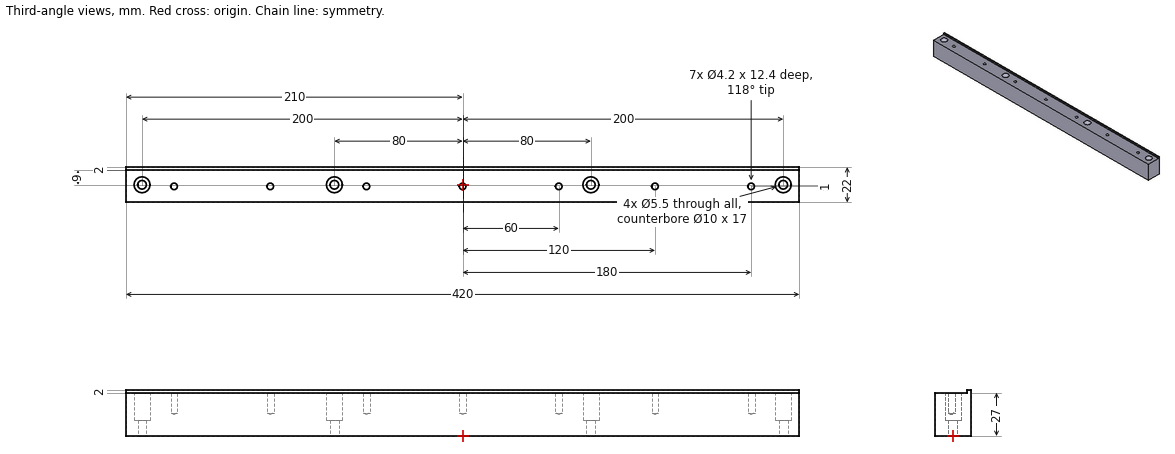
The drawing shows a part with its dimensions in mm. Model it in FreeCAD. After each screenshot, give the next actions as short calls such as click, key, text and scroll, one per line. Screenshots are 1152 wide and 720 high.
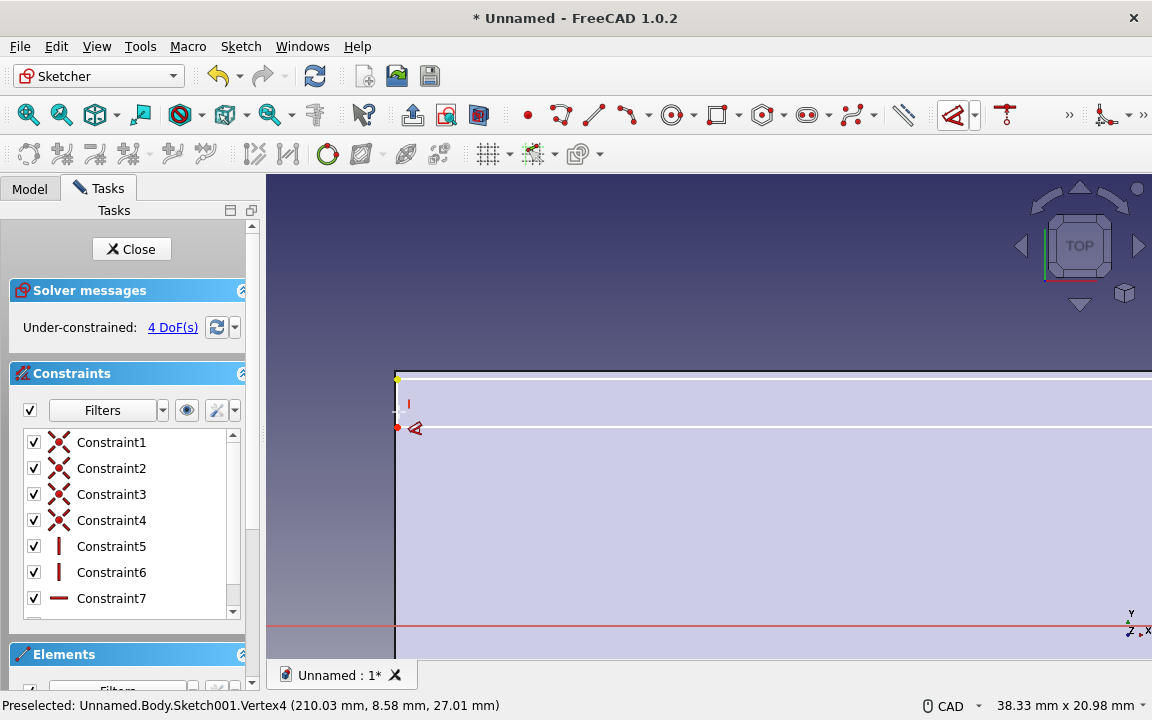
click(397, 403)
click(363, 403)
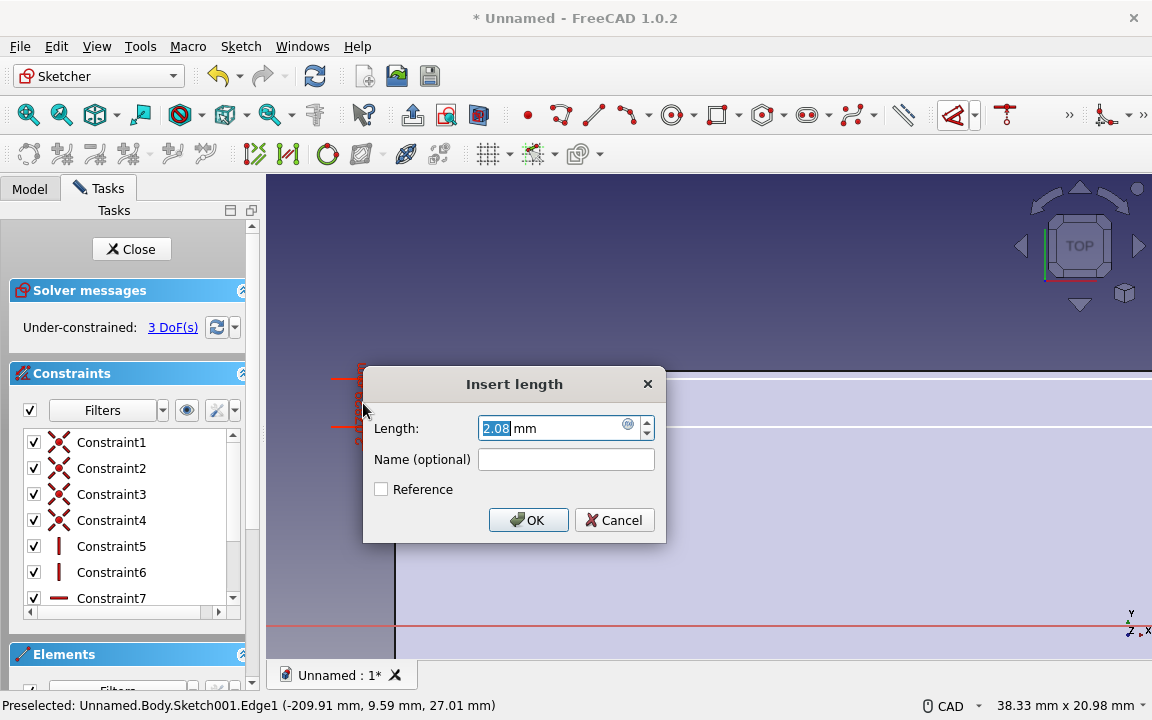
text(2)
key(Return)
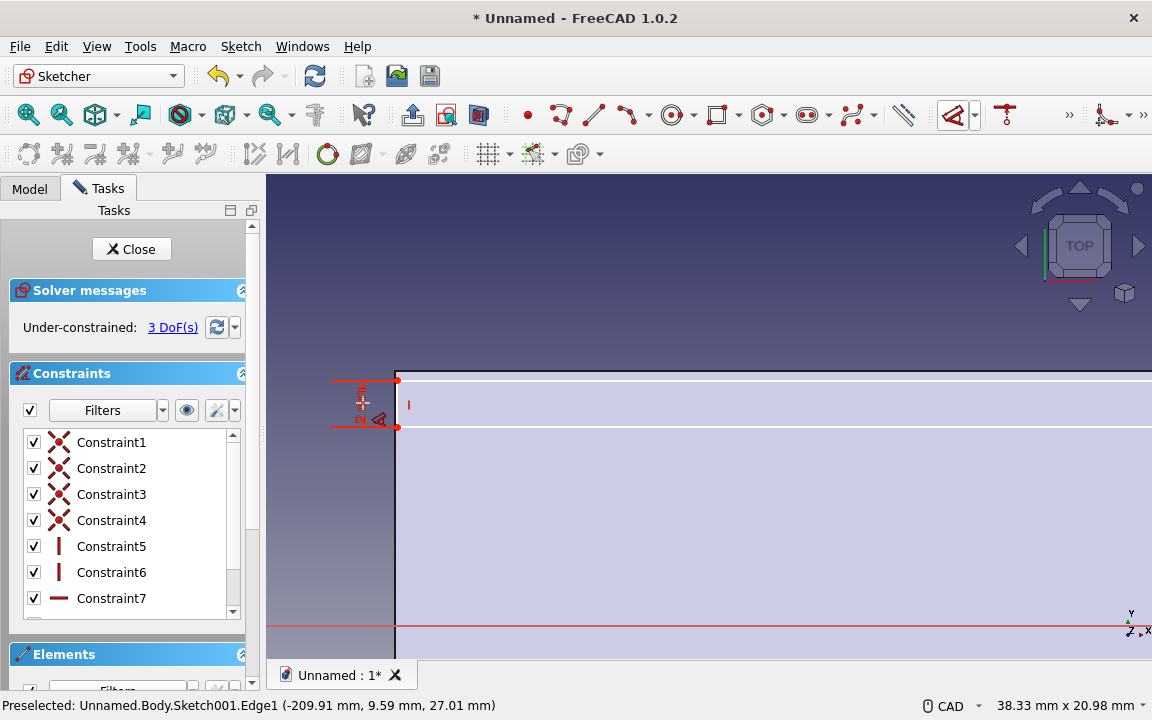
scroll(399, 412, down, 15)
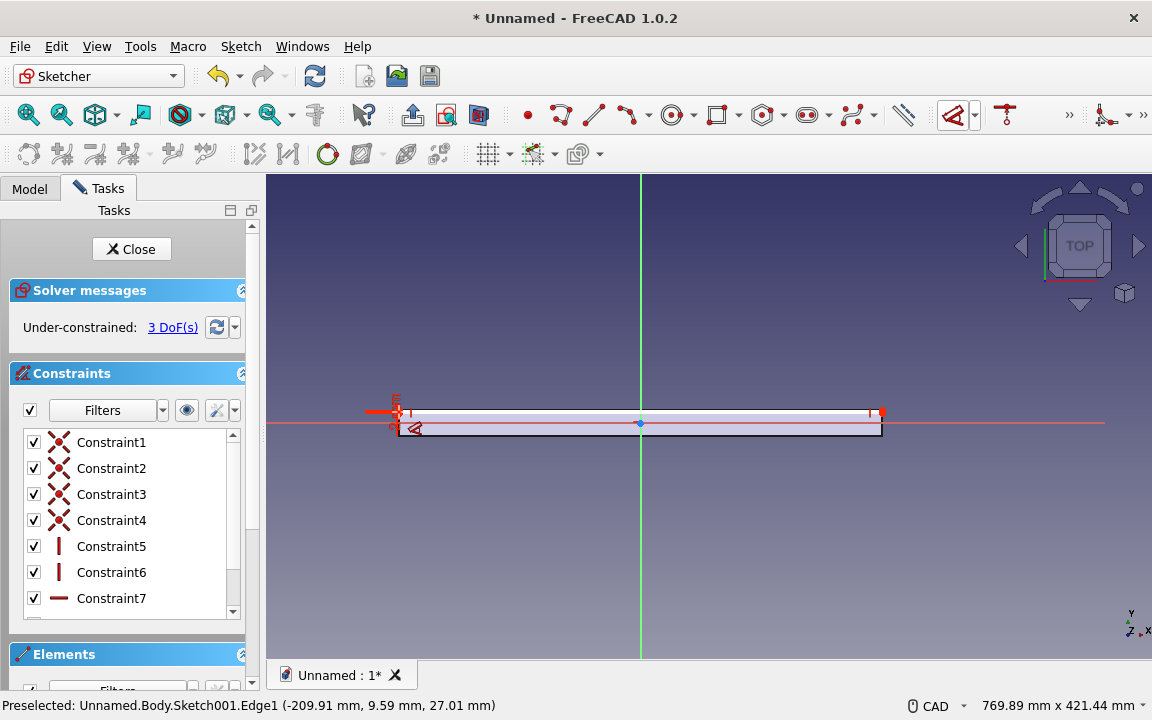
scroll(399, 413, up, 9)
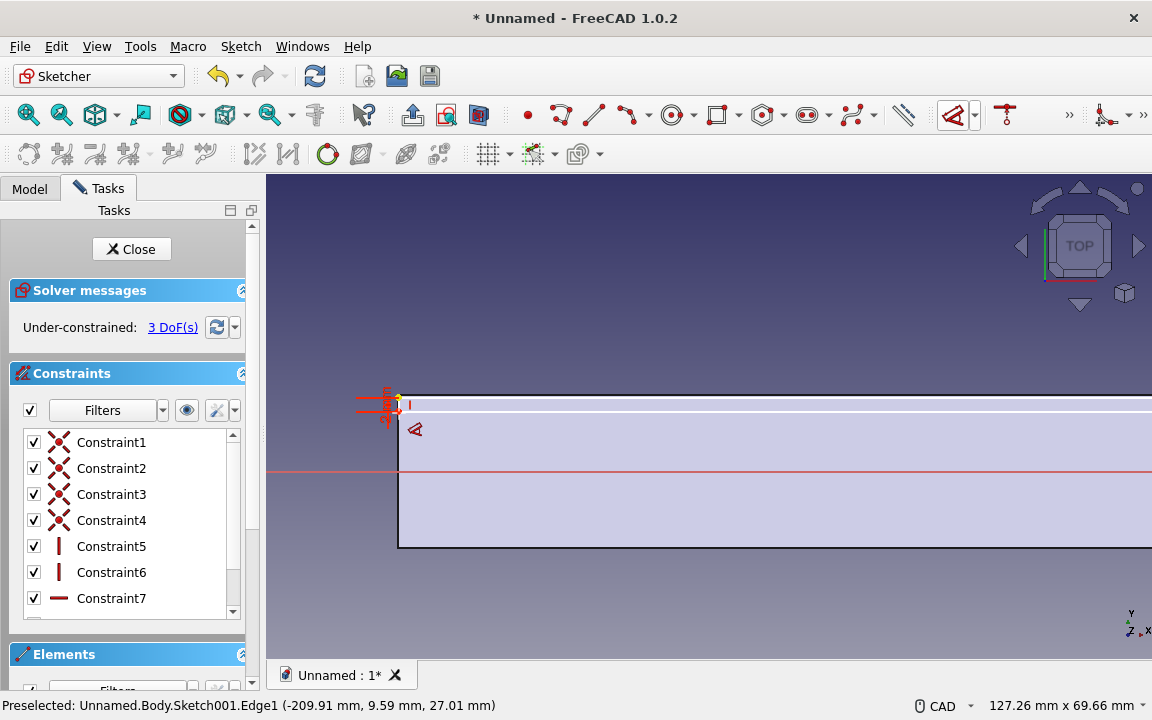
click(399, 412)
click(365, 442)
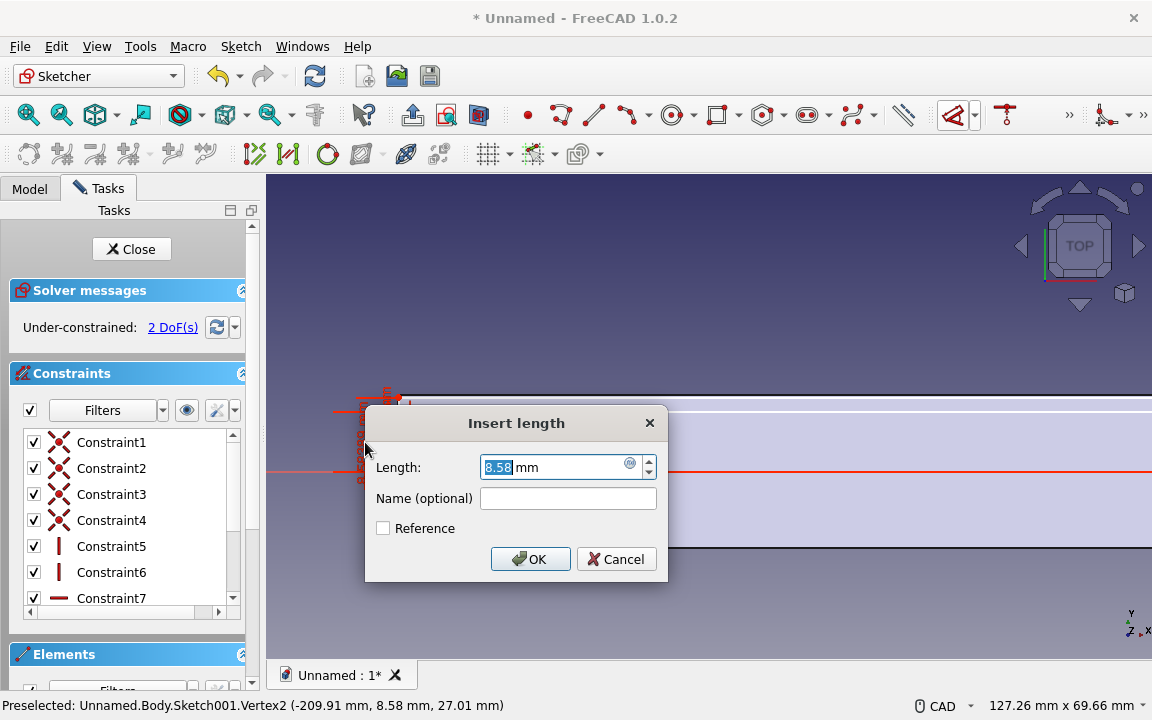
text(9)
key(Return)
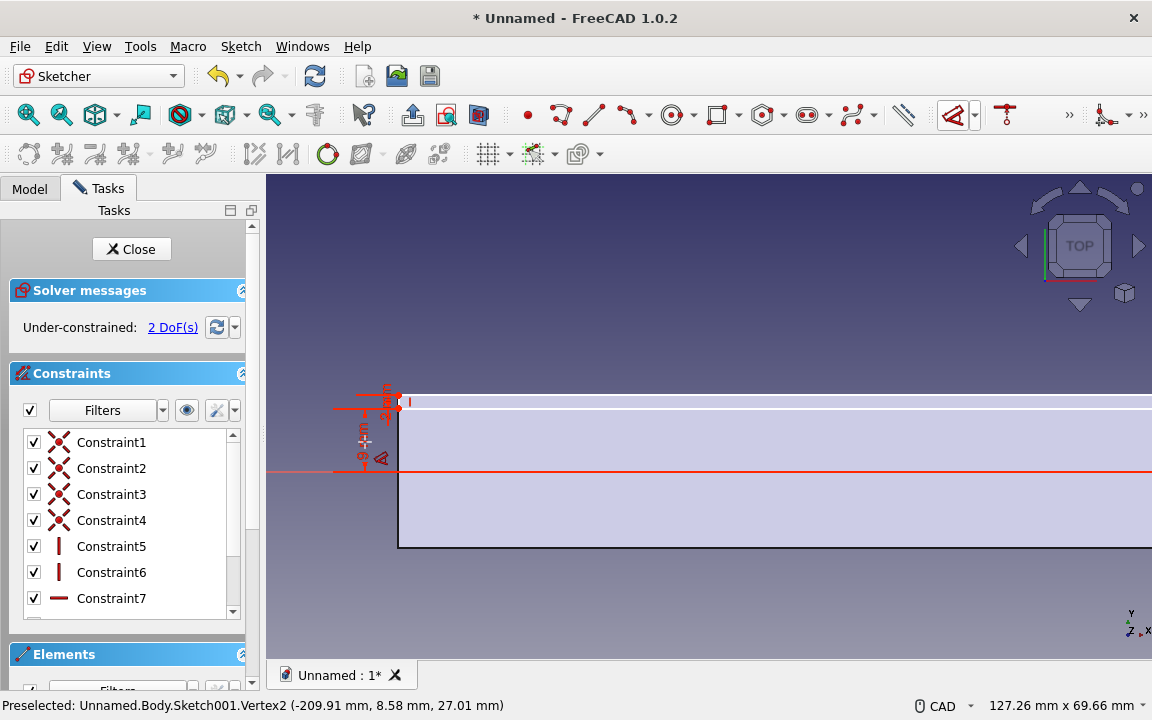
click(983, 409)
click(693, 375)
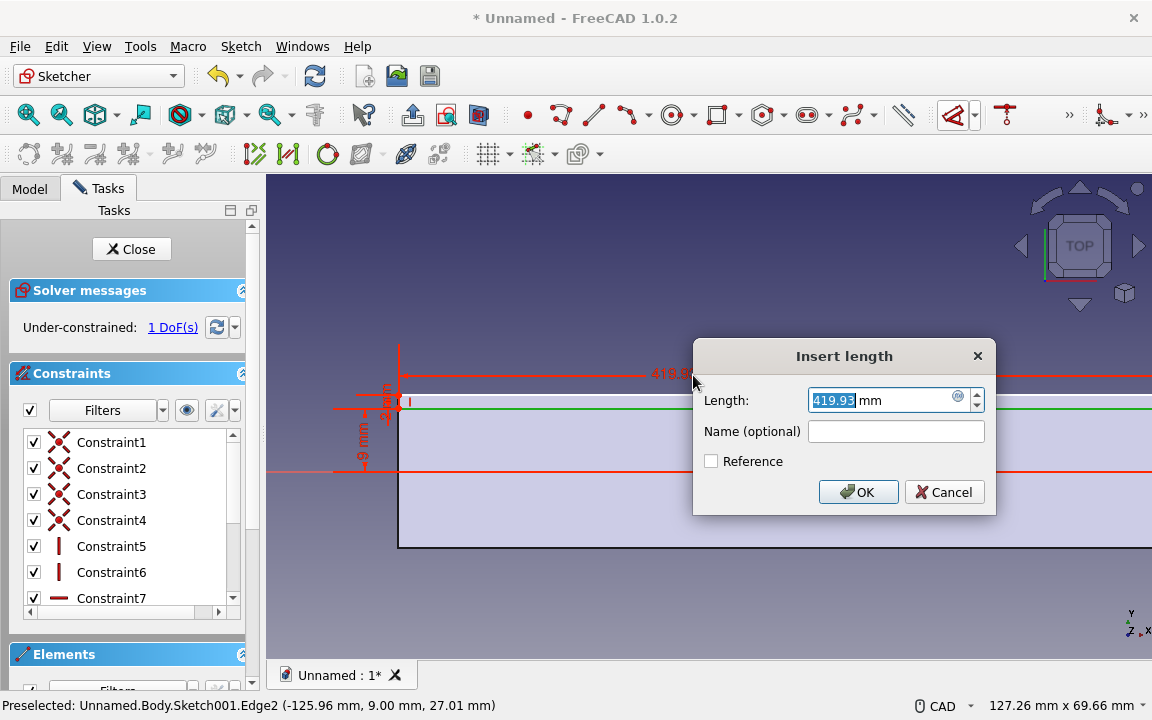
text(420)
key(Return)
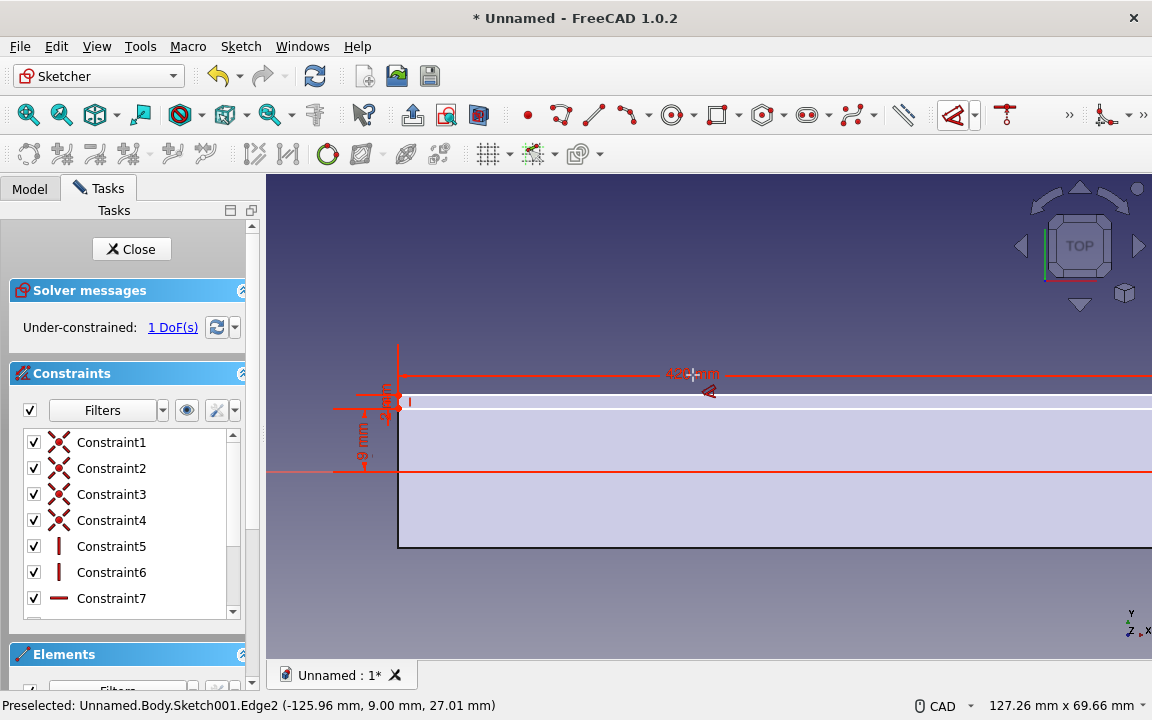
click(398, 395)
click(693, 506)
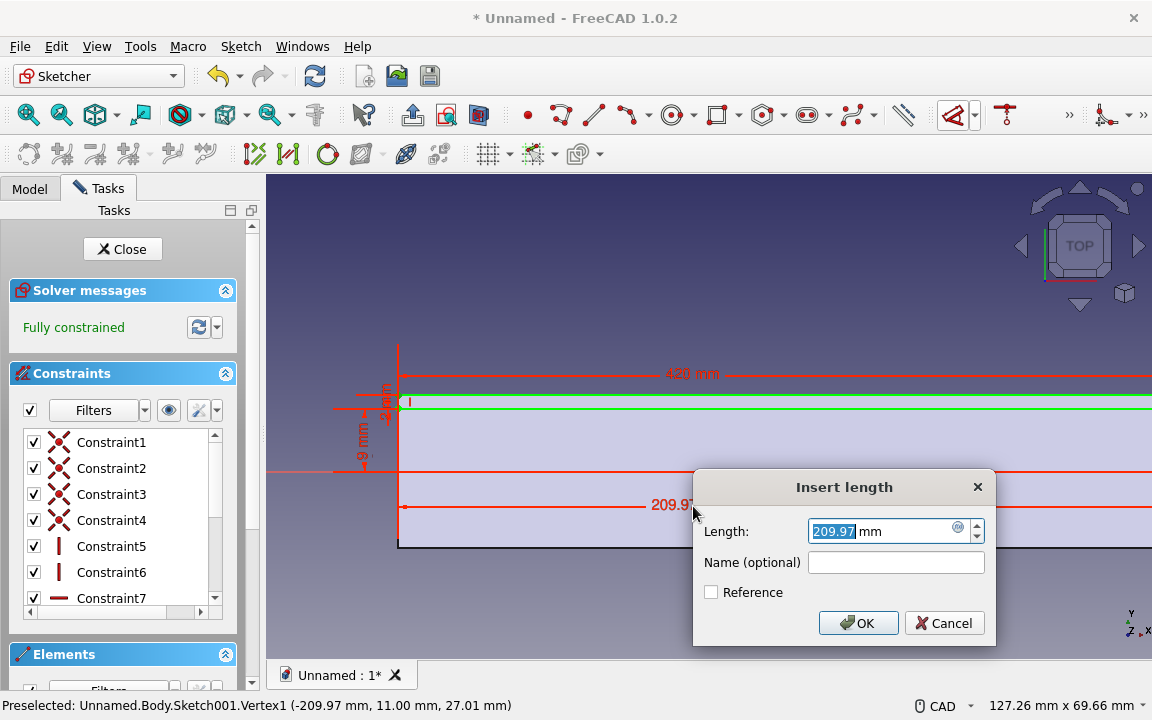
text(210)
key(Return)
key(Escape)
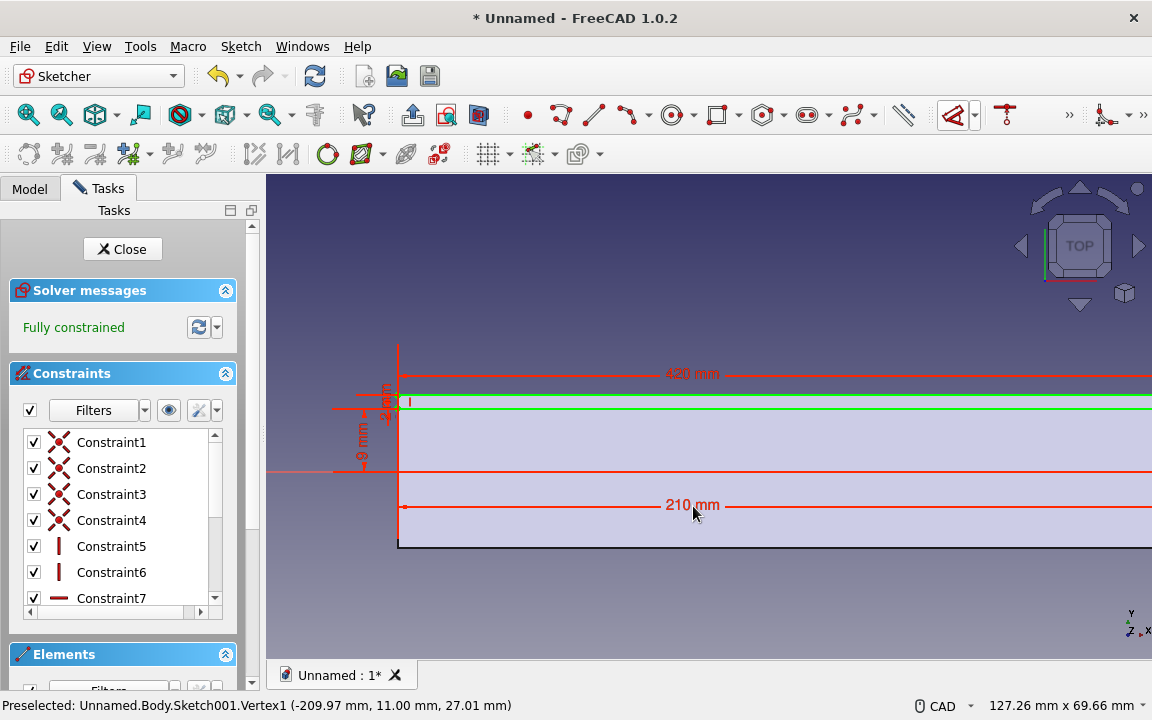
click(123, 249)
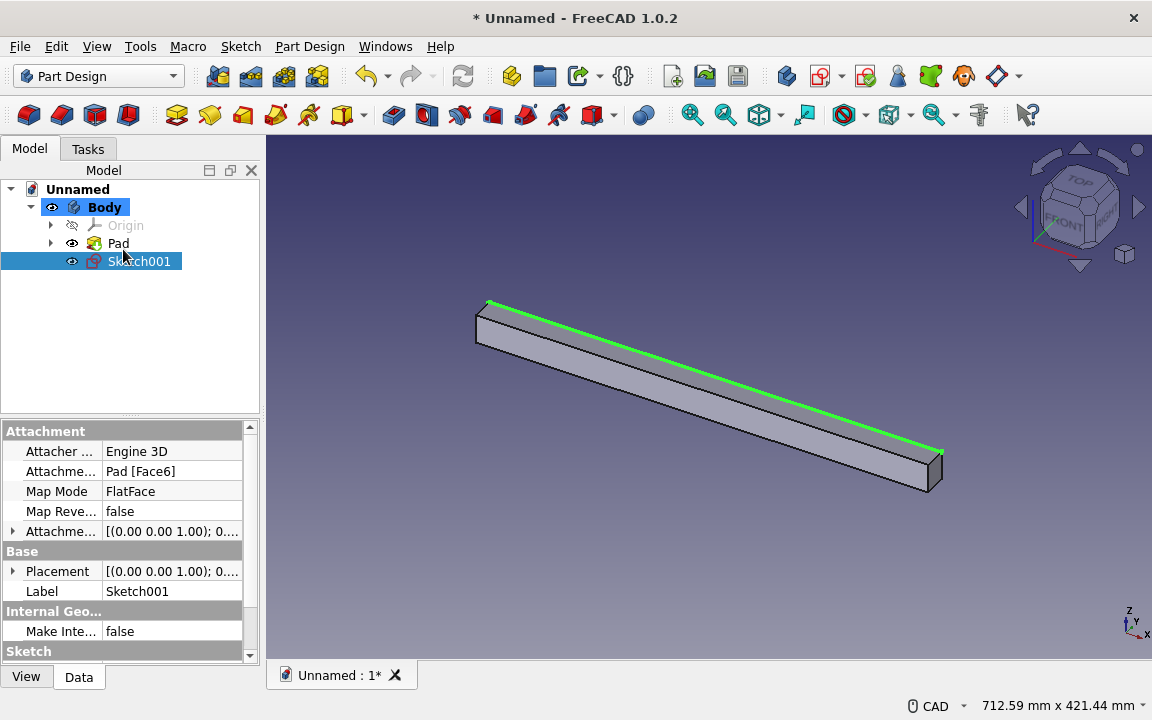
click(177, 116)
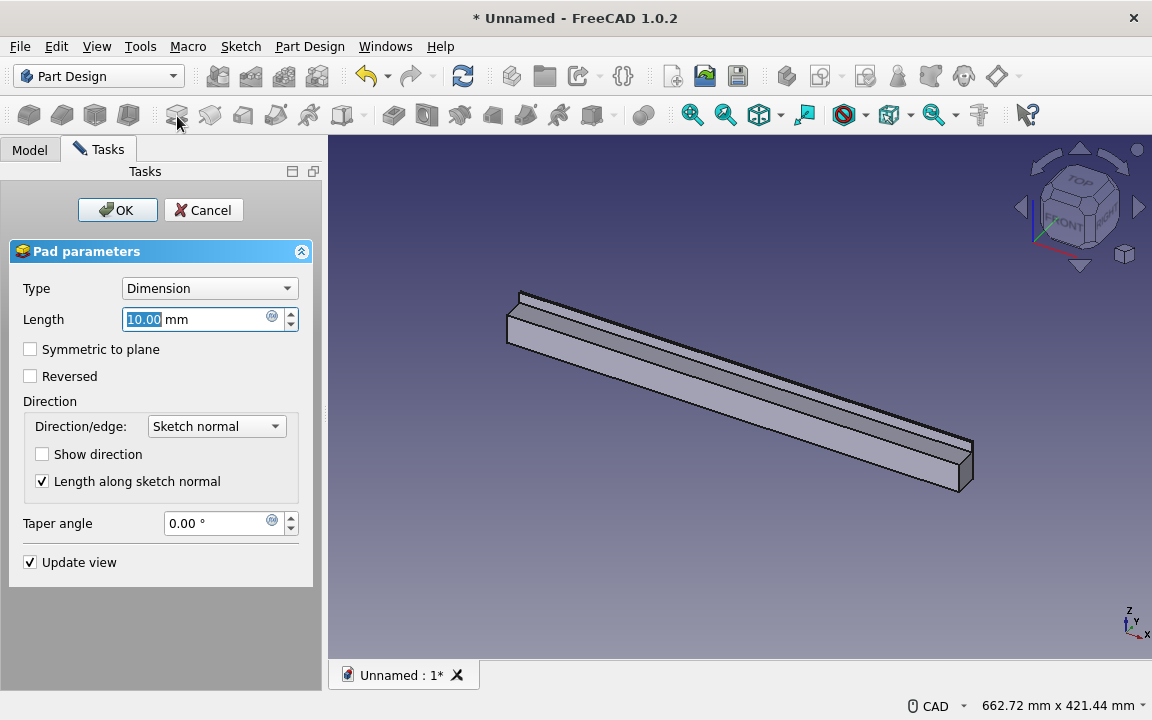
text(2)
key(Tab)